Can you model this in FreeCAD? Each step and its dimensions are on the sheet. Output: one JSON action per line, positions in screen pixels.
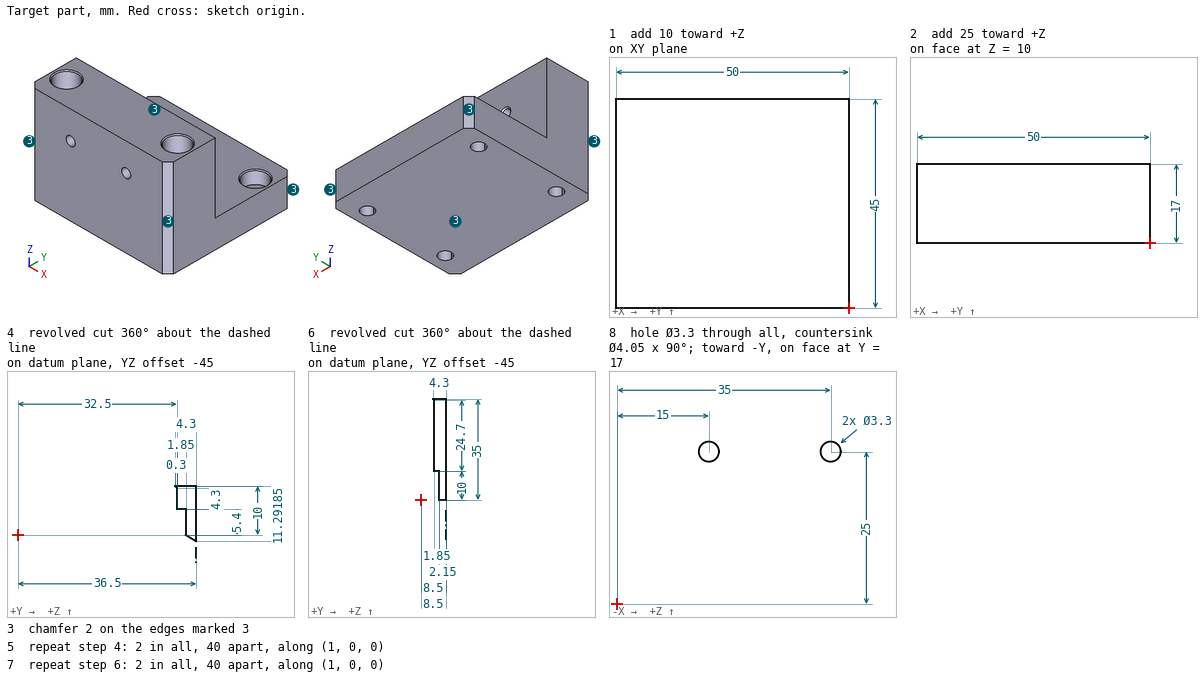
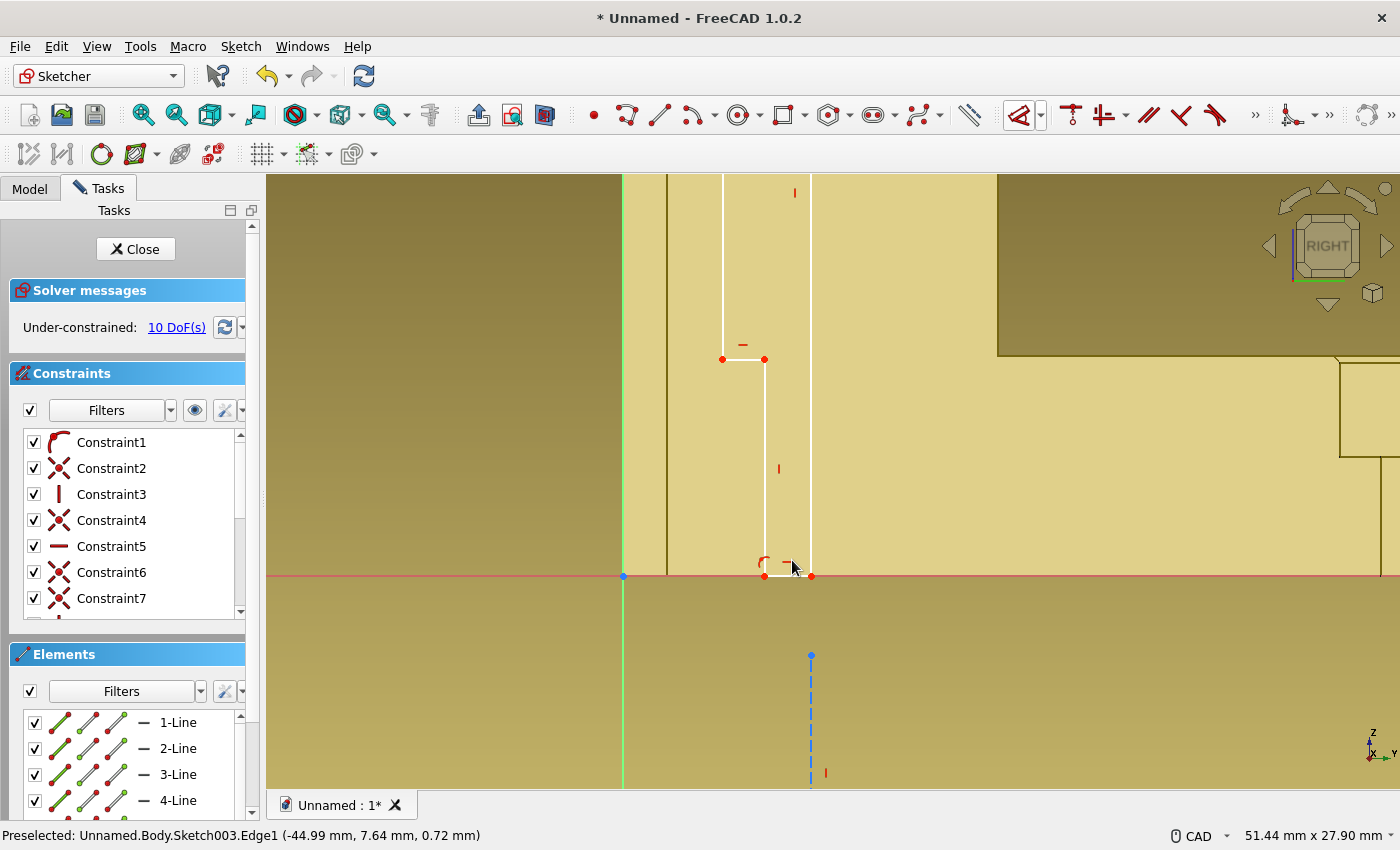
{"action": "left_click", "coordinate": [811, 346]}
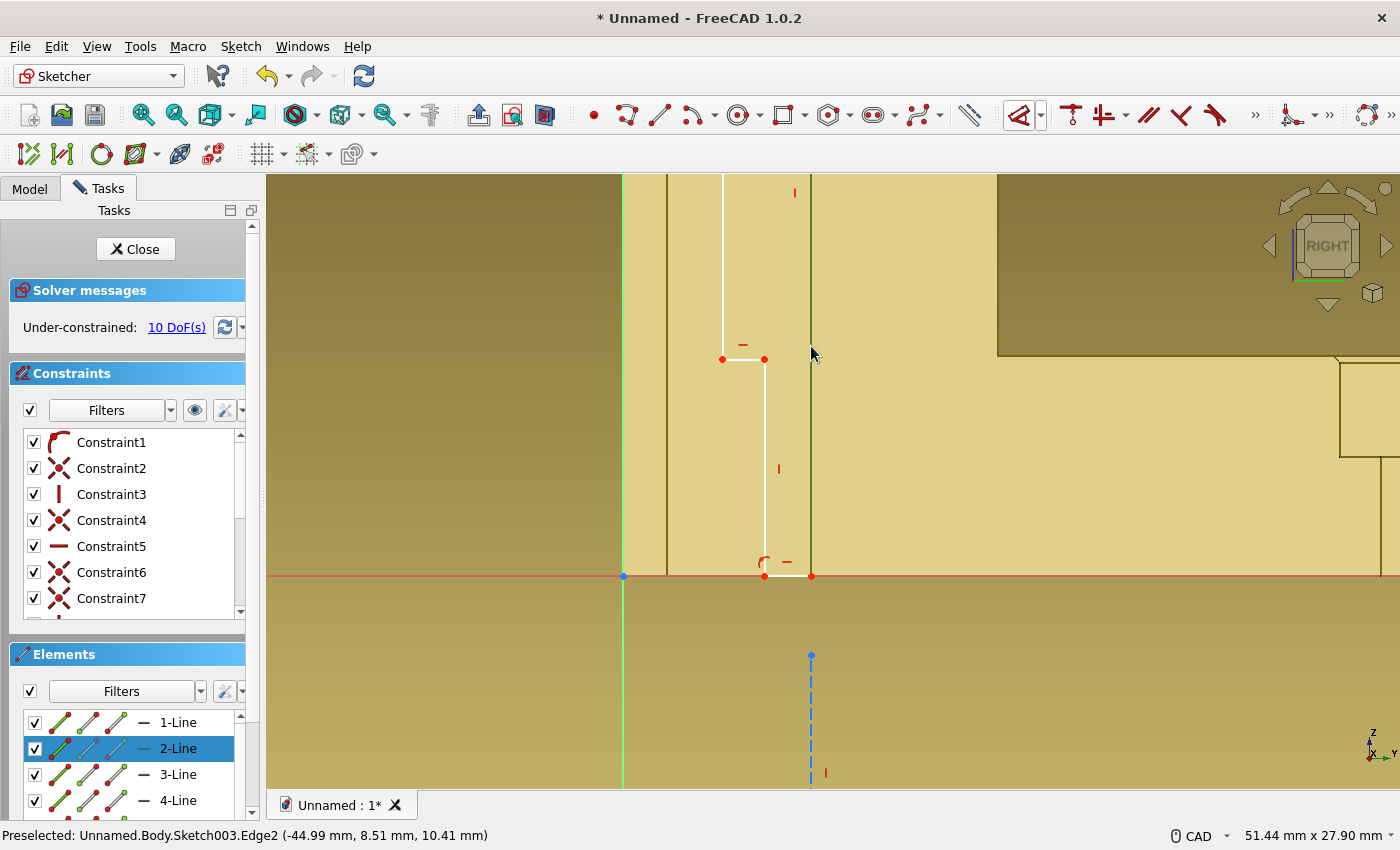
{"action": "key", "text": "i"}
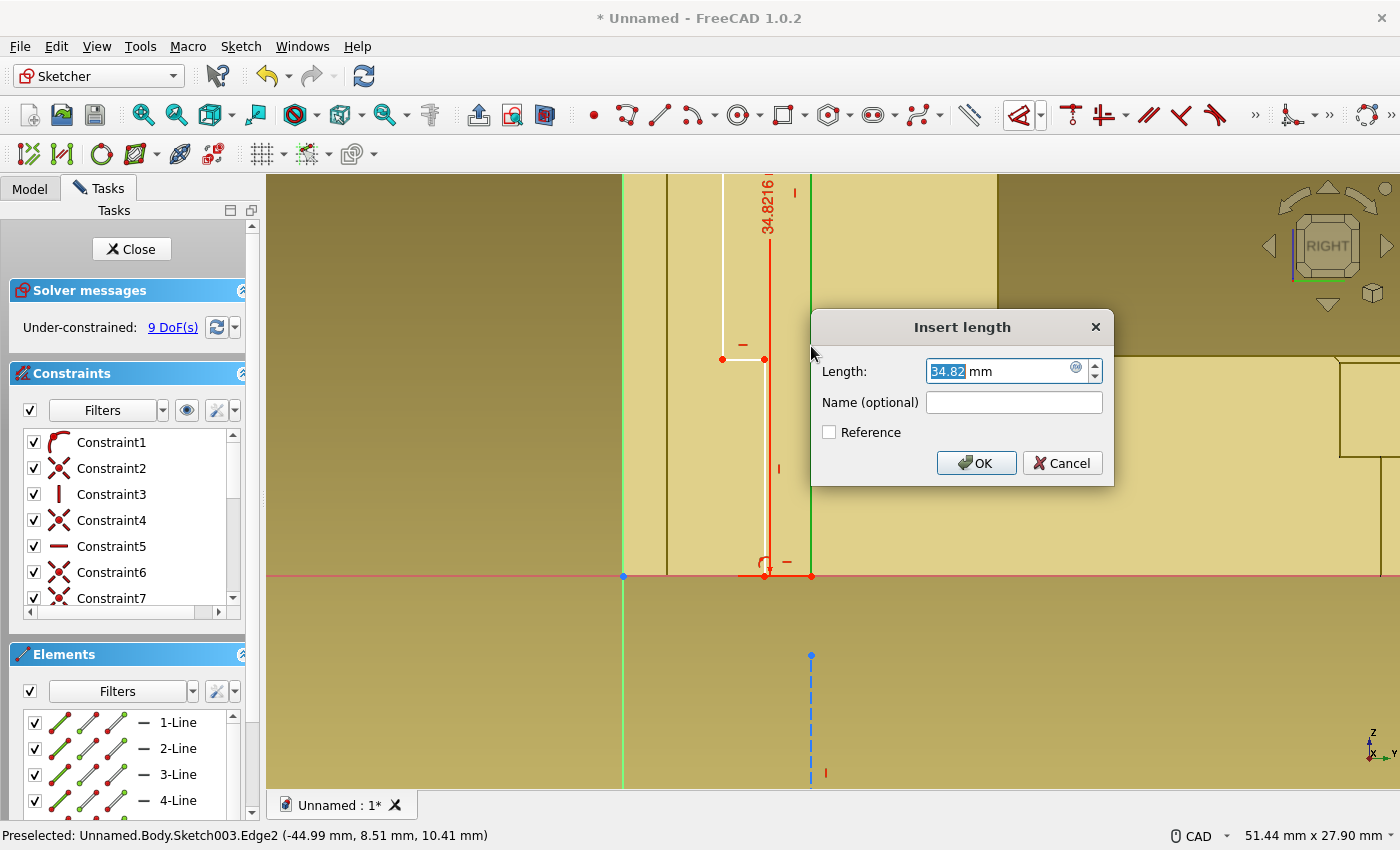
{"action": "type", "text": "35"}
{"action": "key", "text": "Return"}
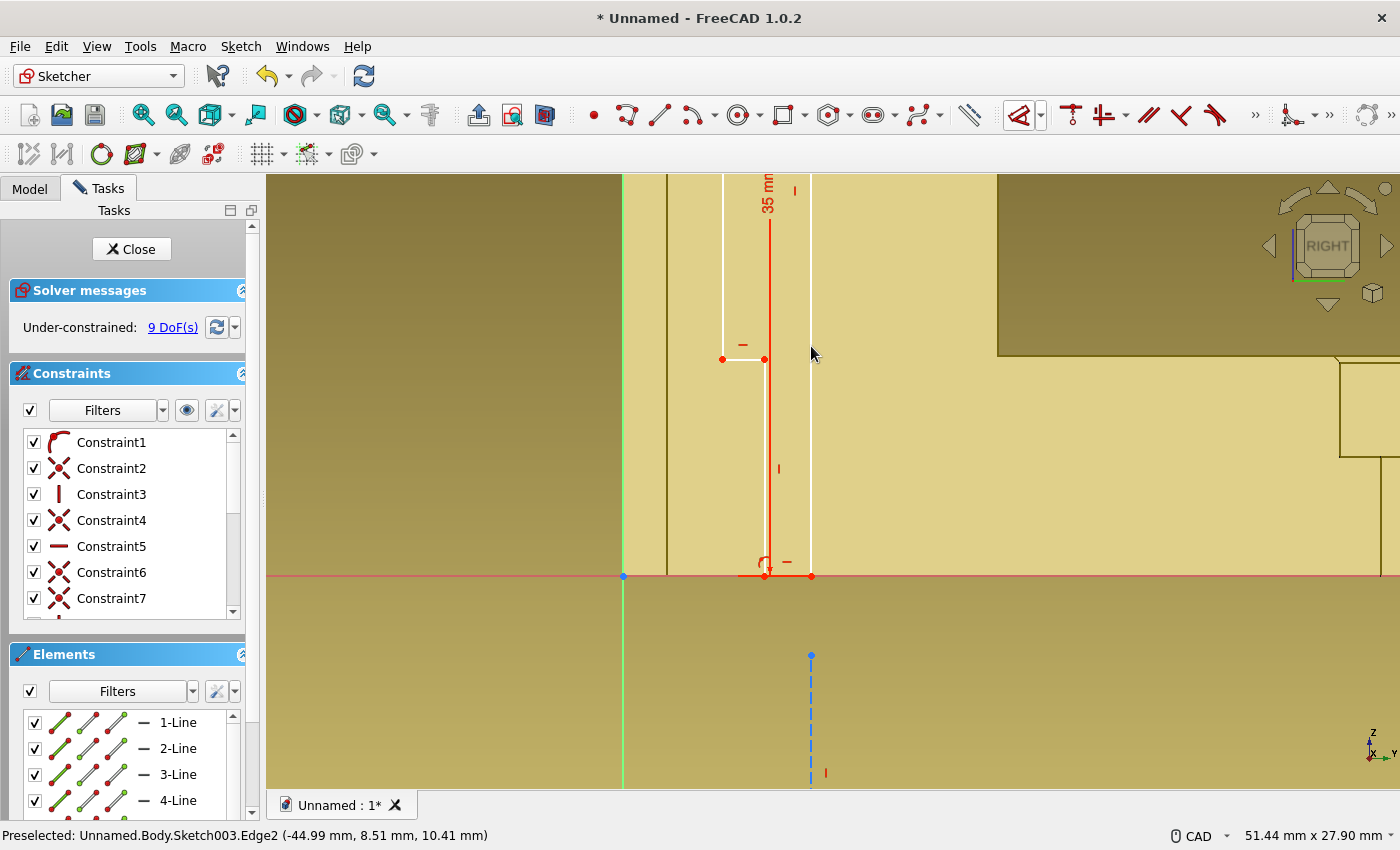
{"action": "left_click", "coordinate": [765, 425]}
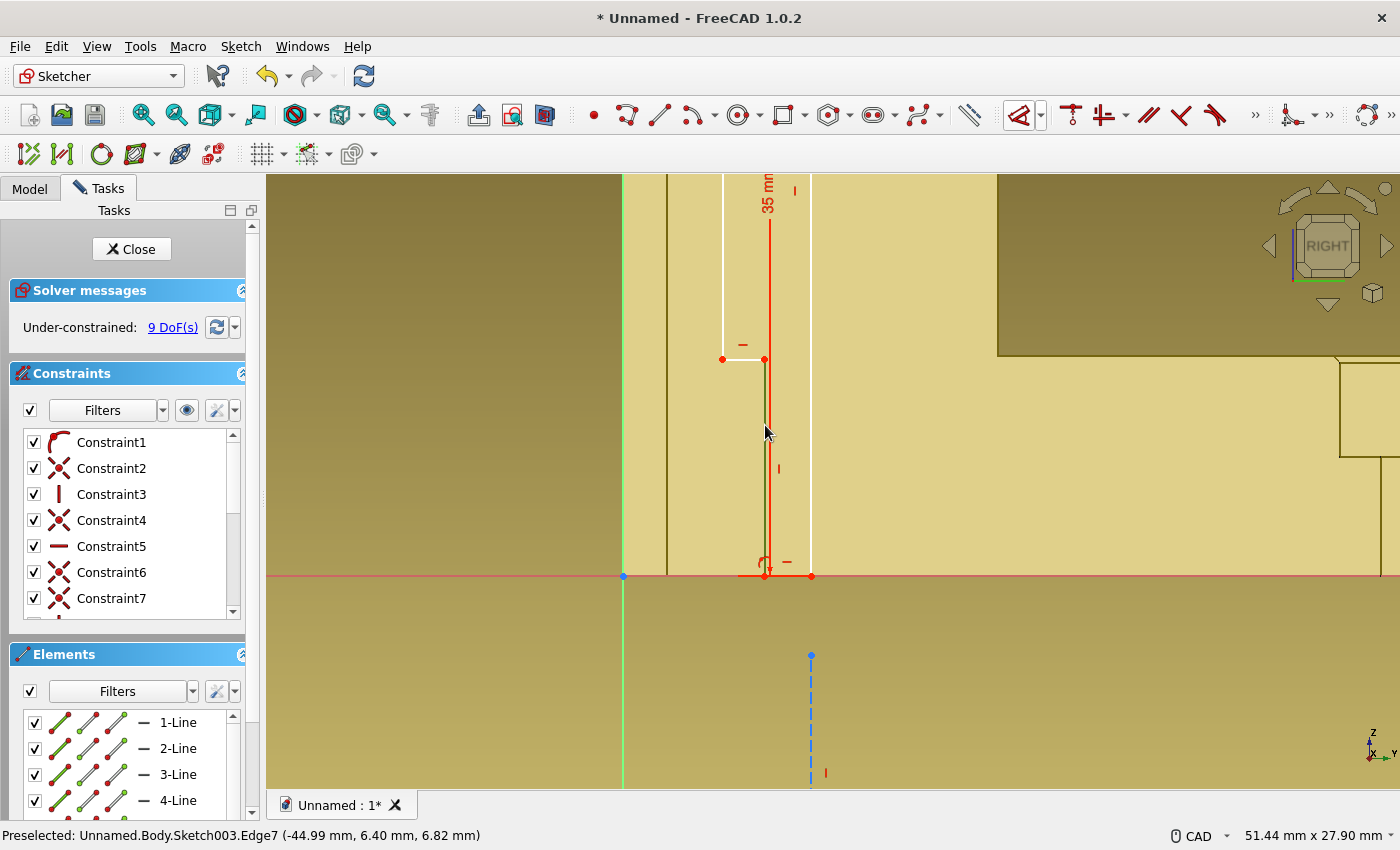
{"action": "key", "text": "i"}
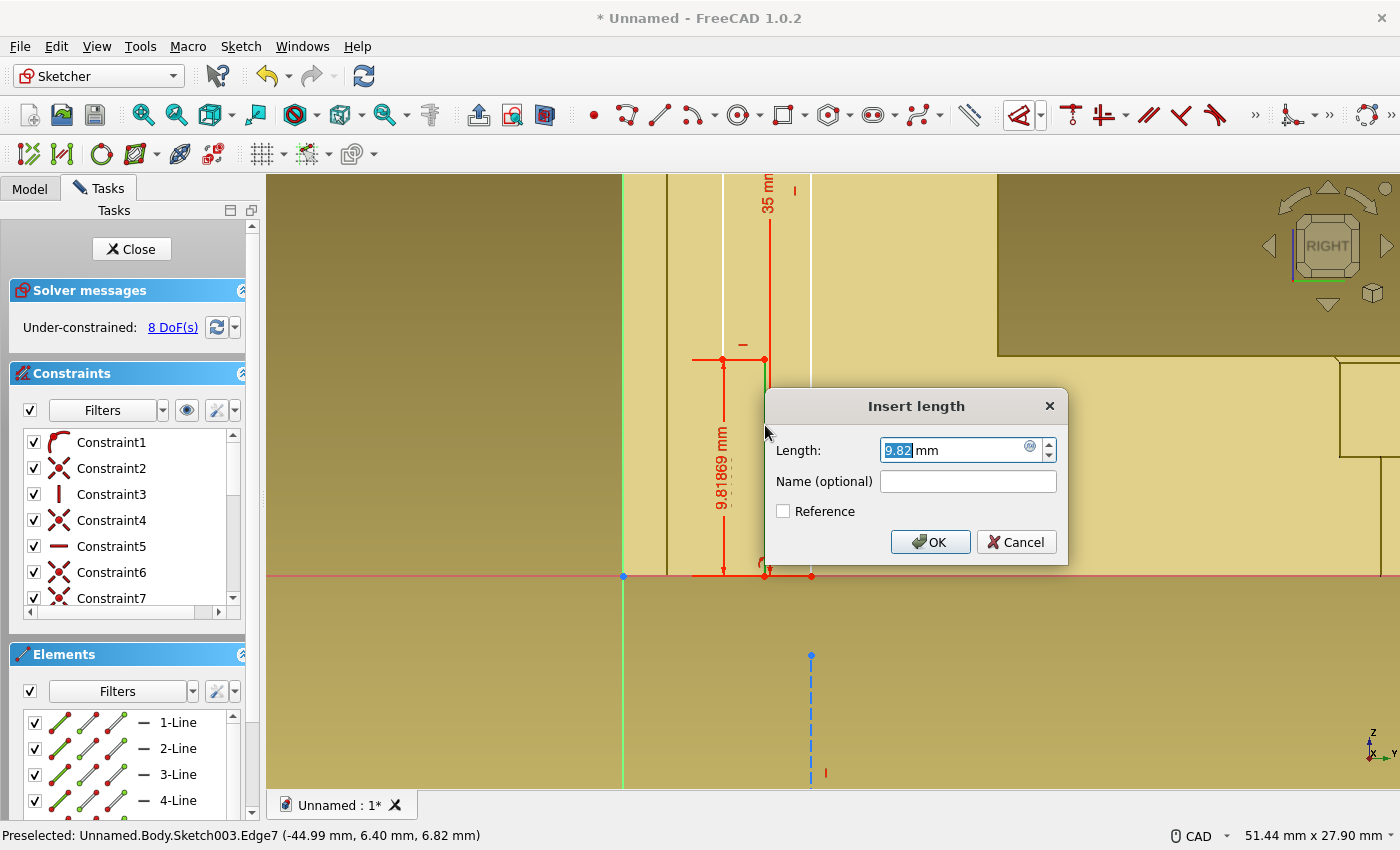
{"action": "type", "text": "10"}
{"action": "key", "text": "Return"}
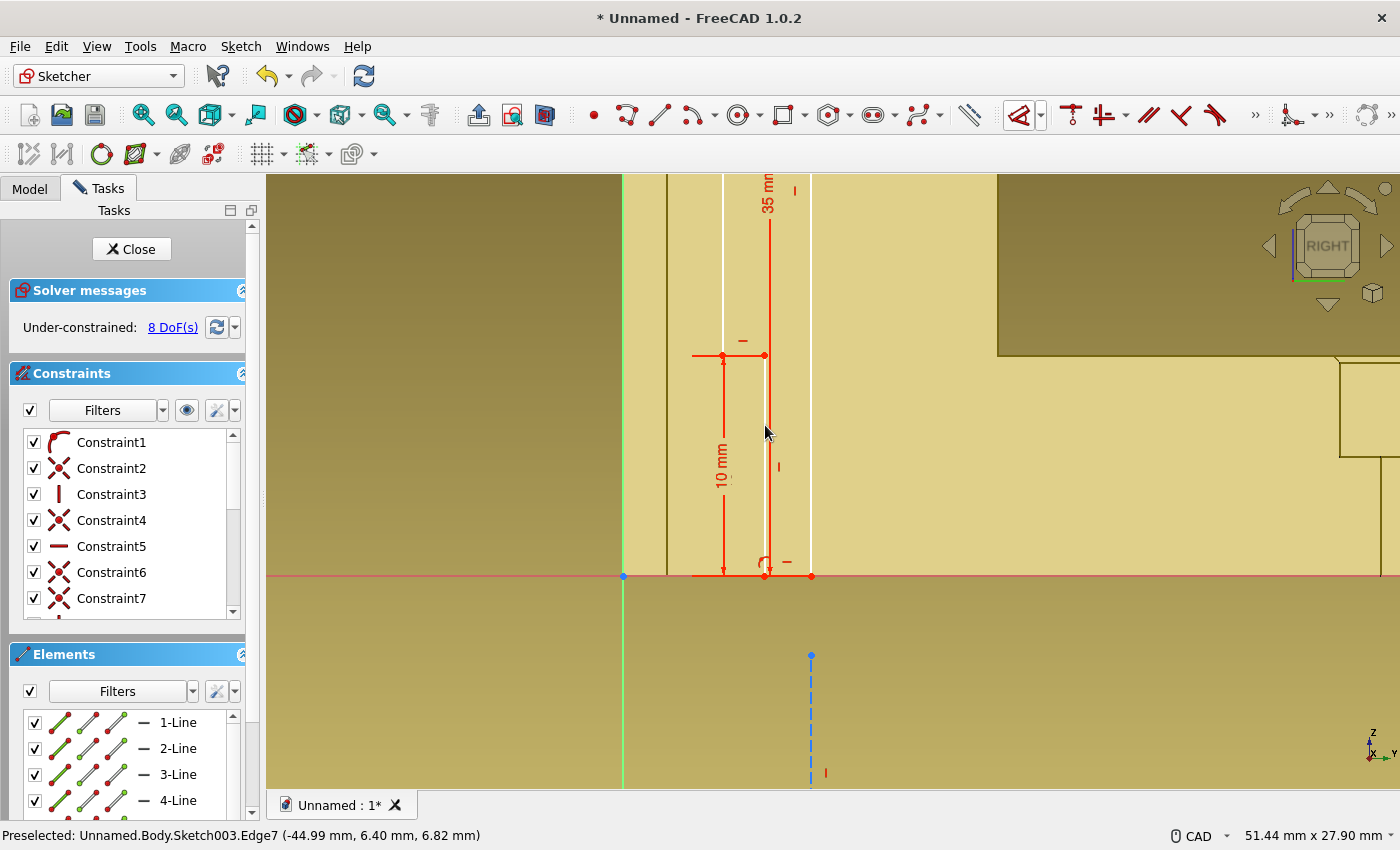
{"action": "scroll", "coordinate": [792, 561], "scroll_direction": "down", "scroll_amount": 5}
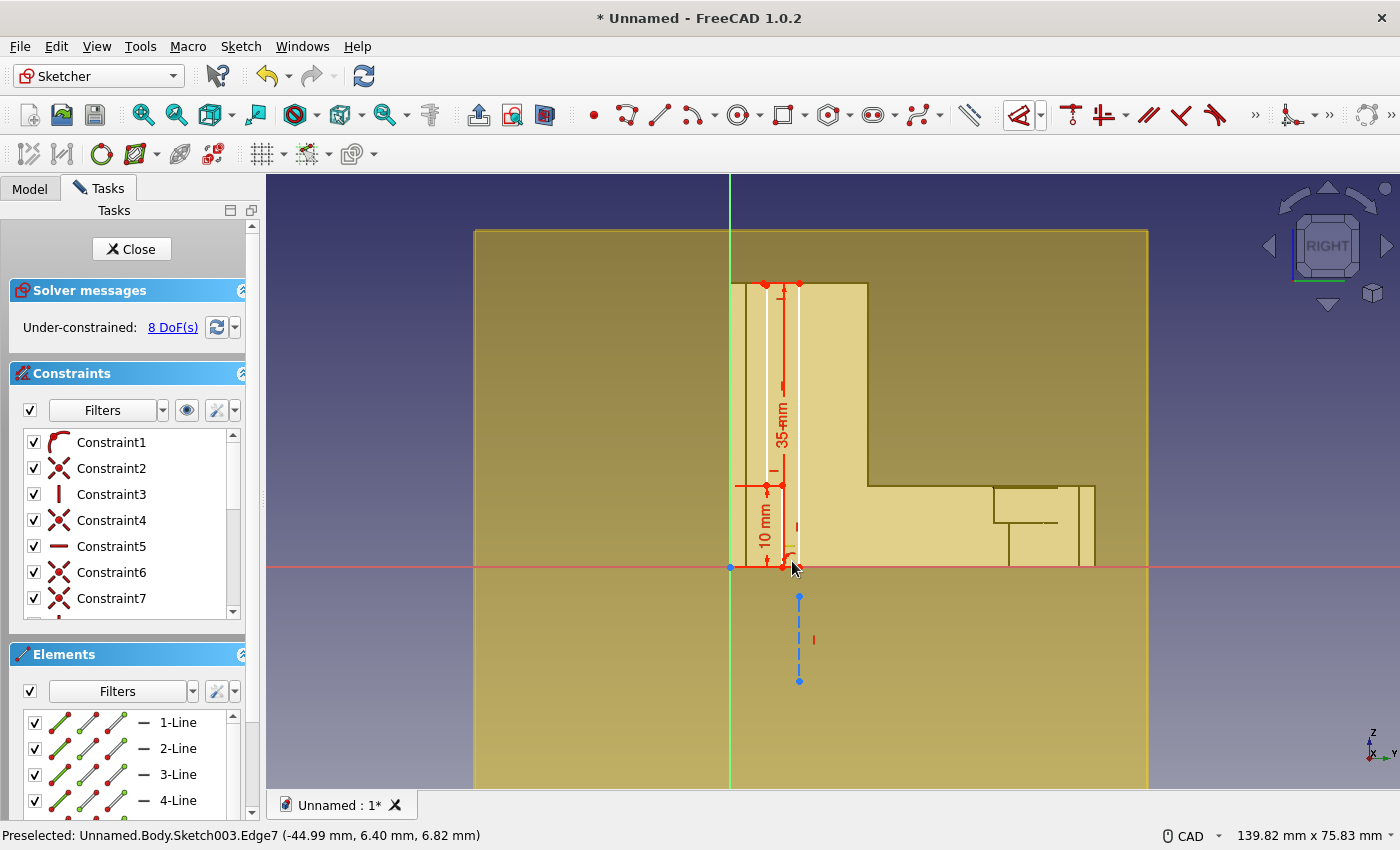
{"action": "scroll", "coordinate": [789, 283], "scroll_direction": "up", "scroll_amount": 2}